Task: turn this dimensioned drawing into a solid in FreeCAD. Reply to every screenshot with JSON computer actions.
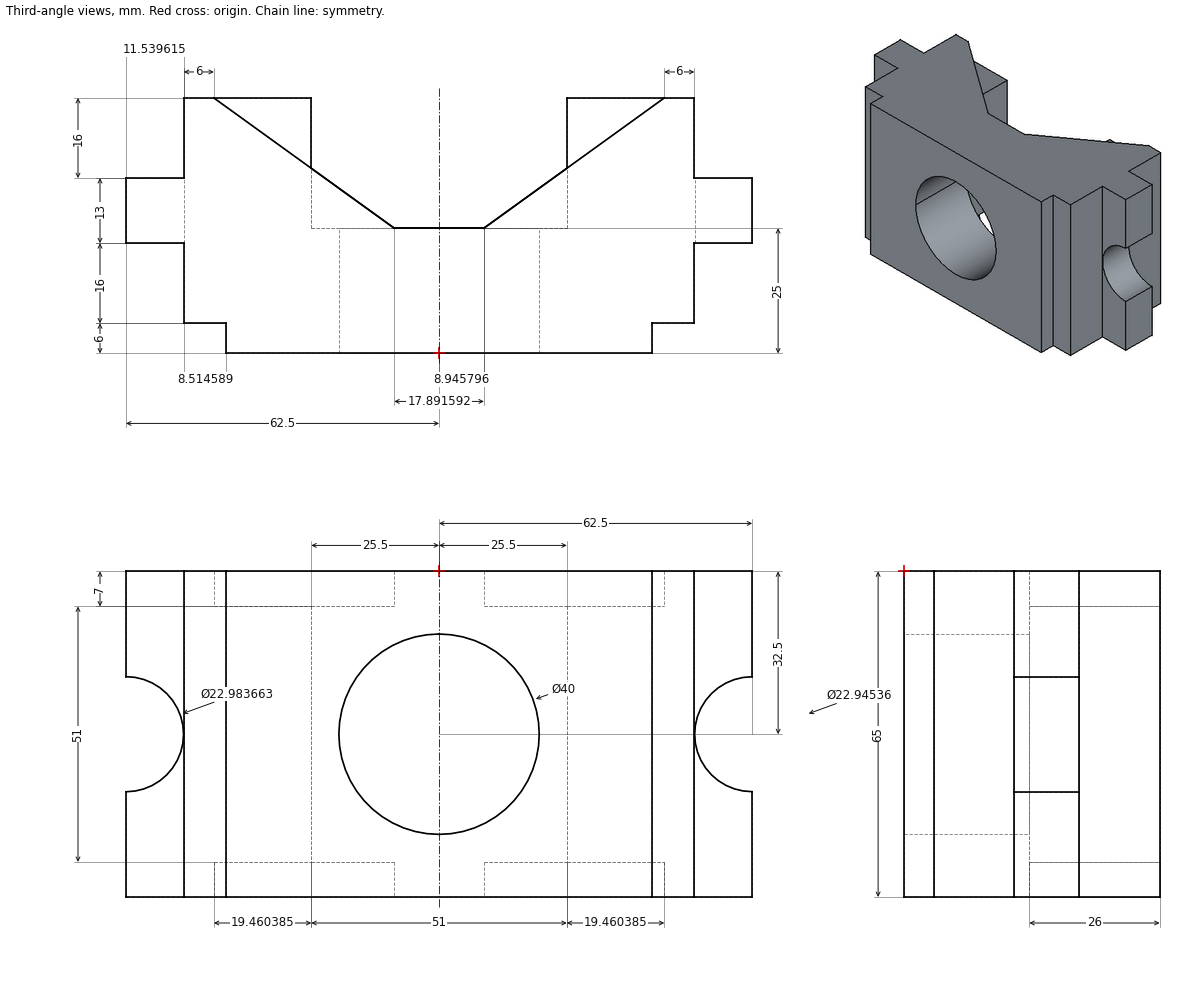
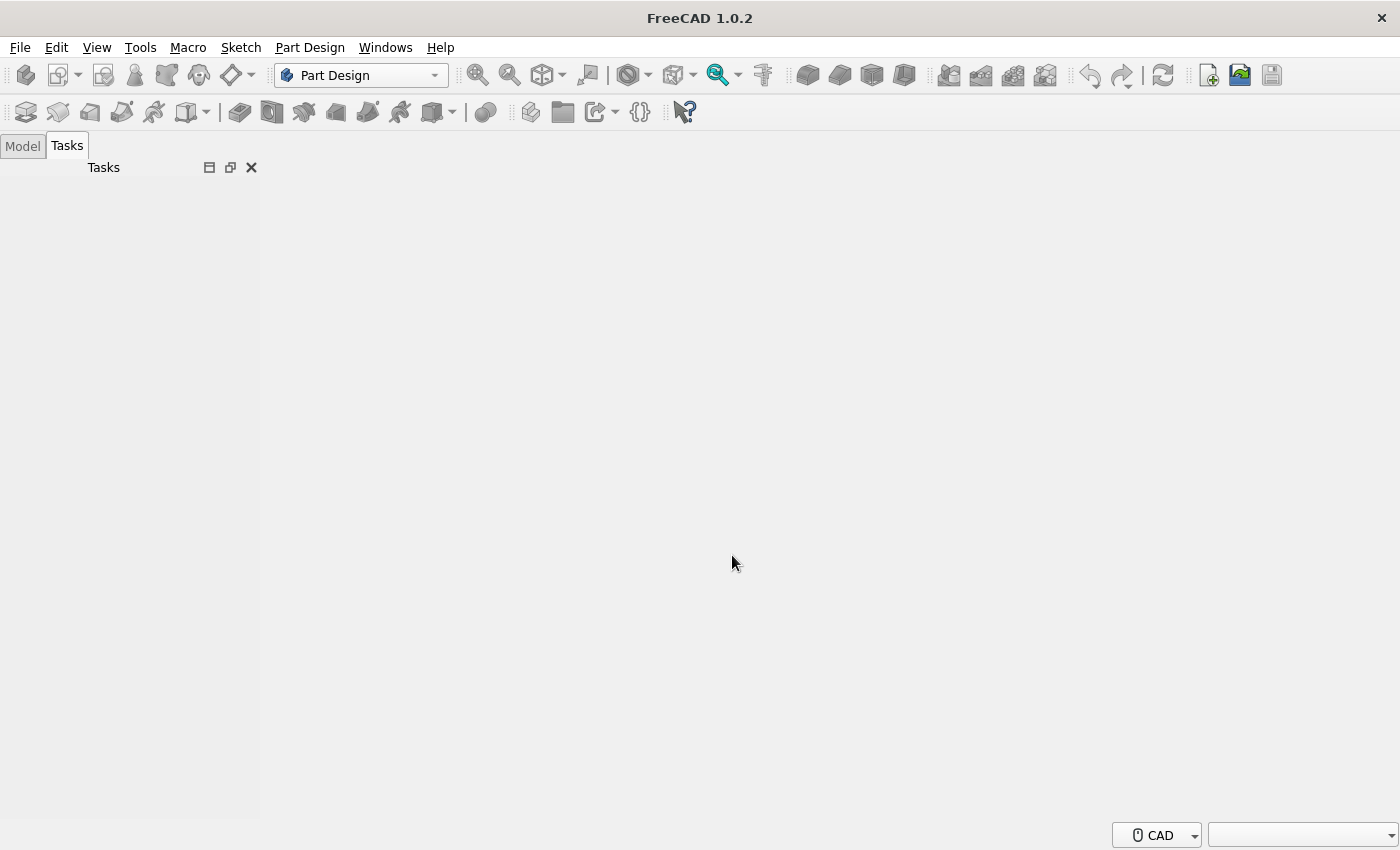
{"action": "left_click", "coordinate": [1208, 76]}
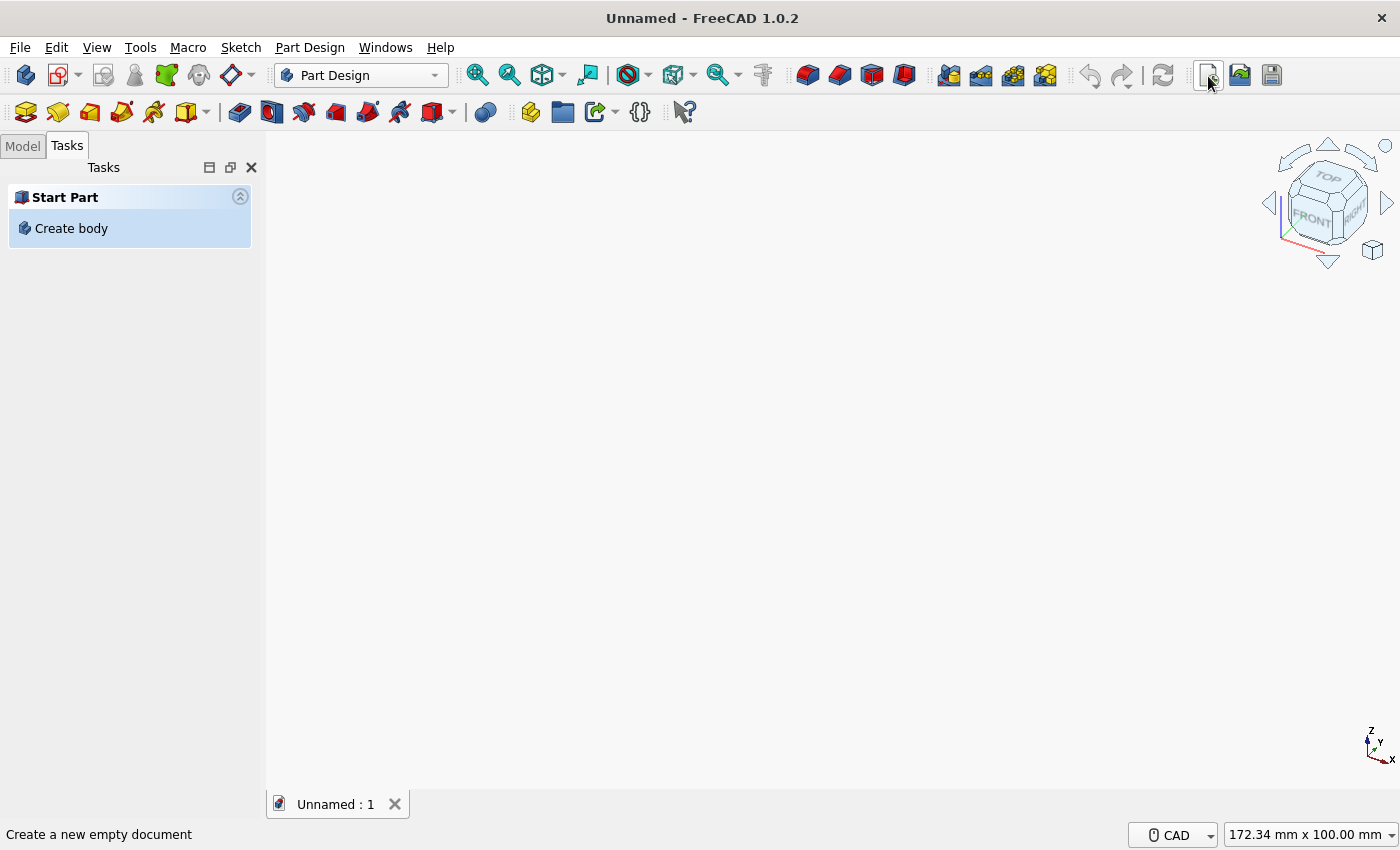
{"action": "left_click", "coordinate": [58, 76]}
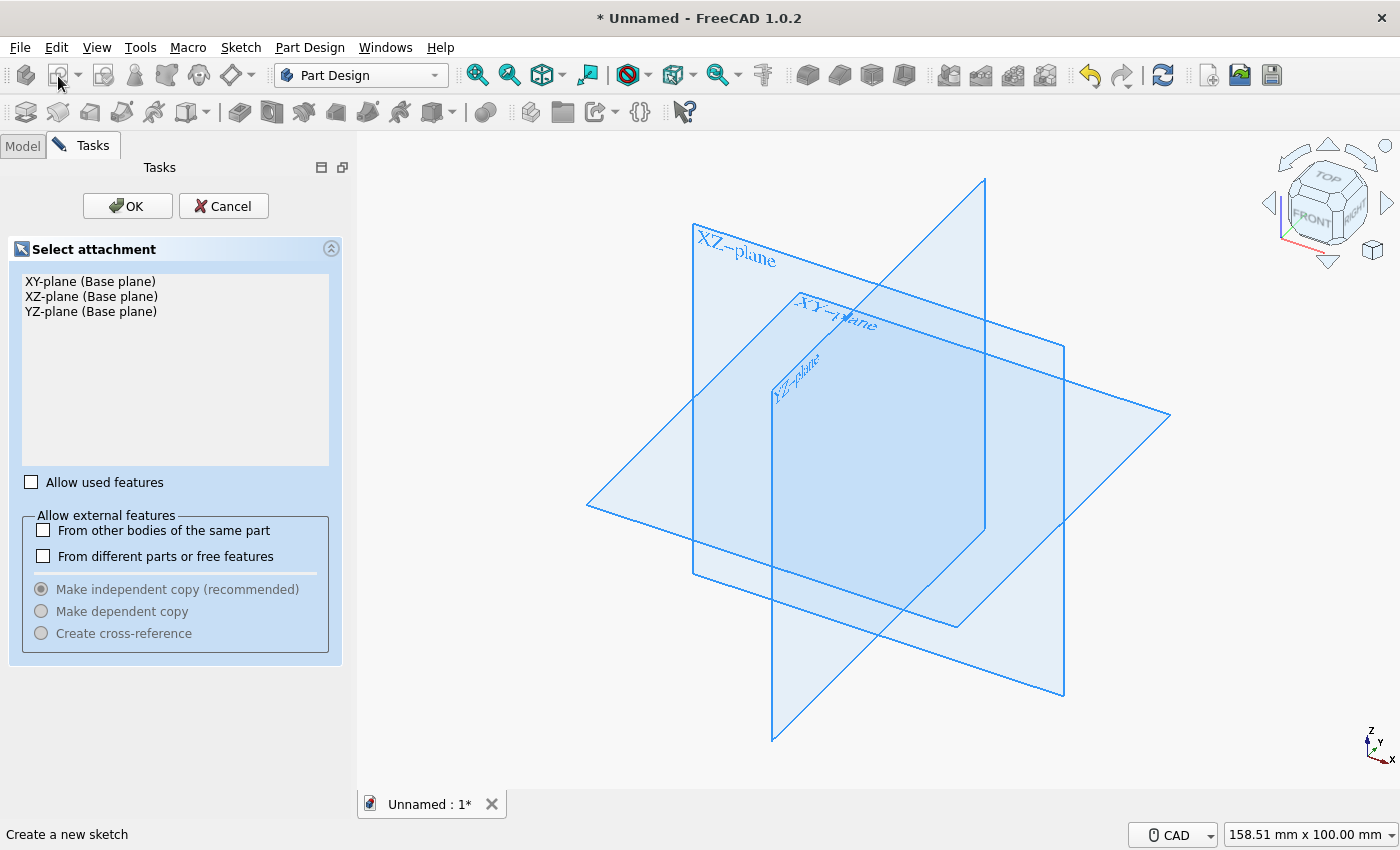
{"action": "left_click", "coordinate": [82, 282]}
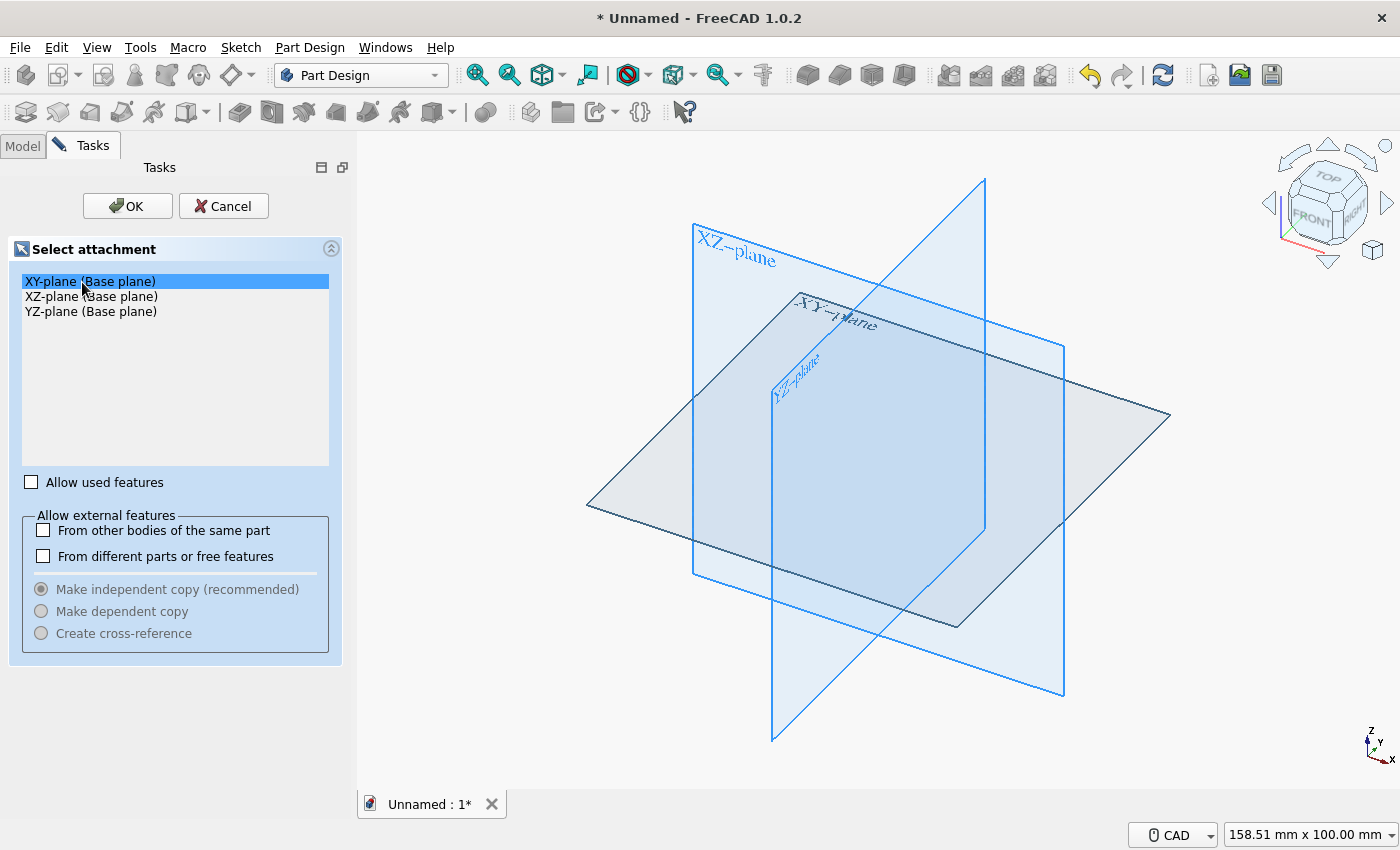
{"action": "left_click", "coordinate": [128, 206]}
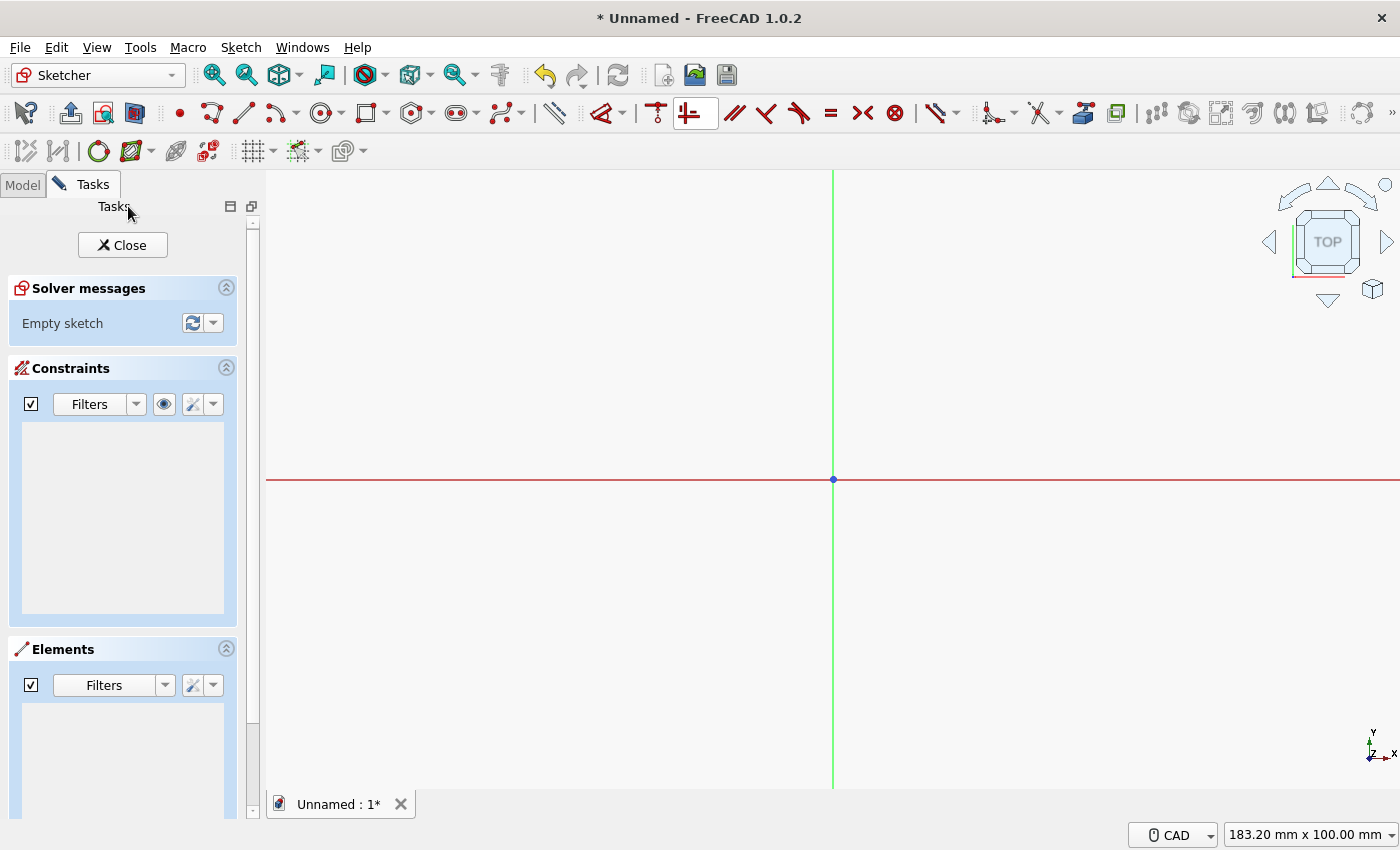
{"action": "scroll", "coordinate": [455, 761], "scroll_direction": "down", "scroll_amount": 1}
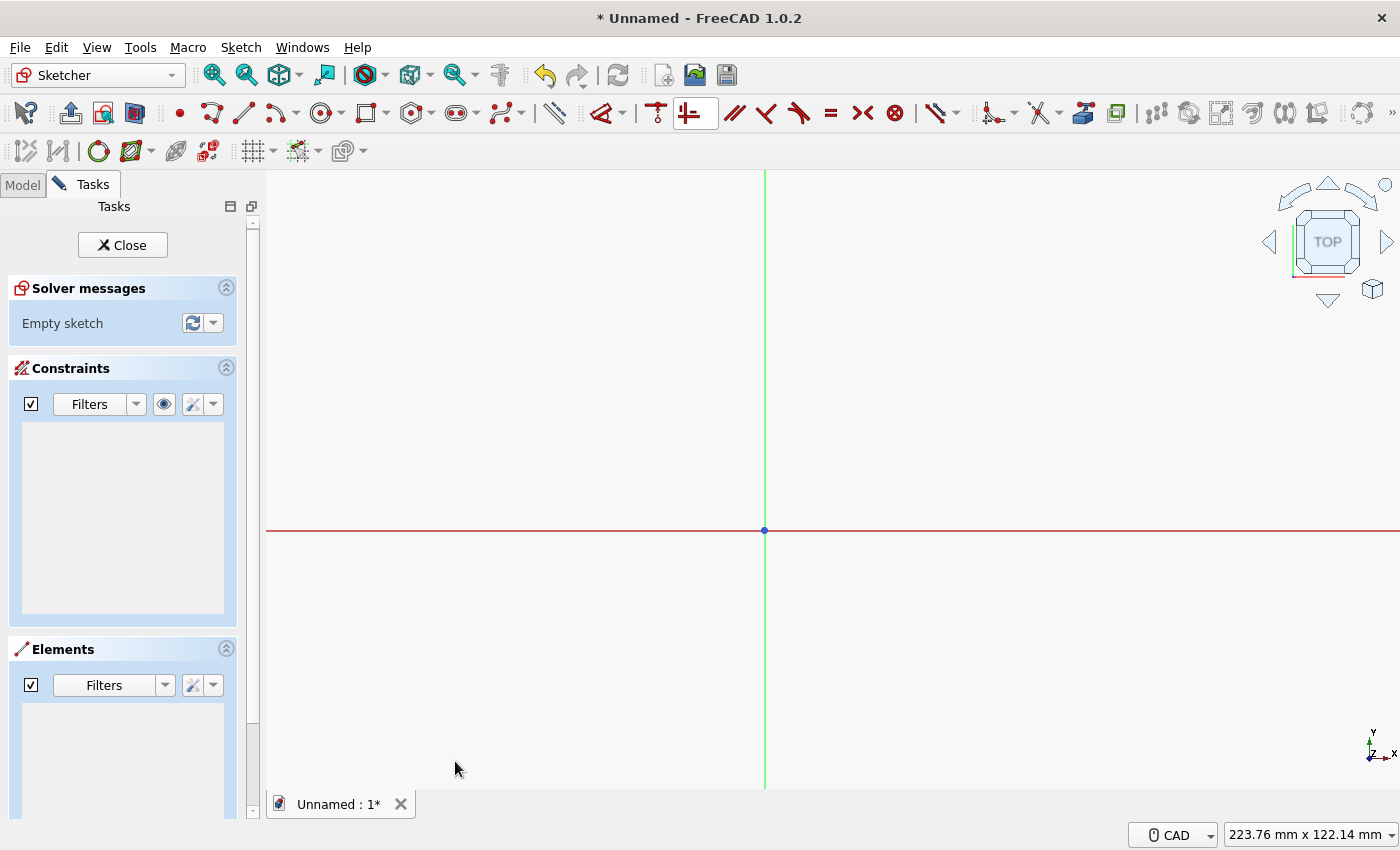
{"action": "left_click", "coordinate": [212, 114]}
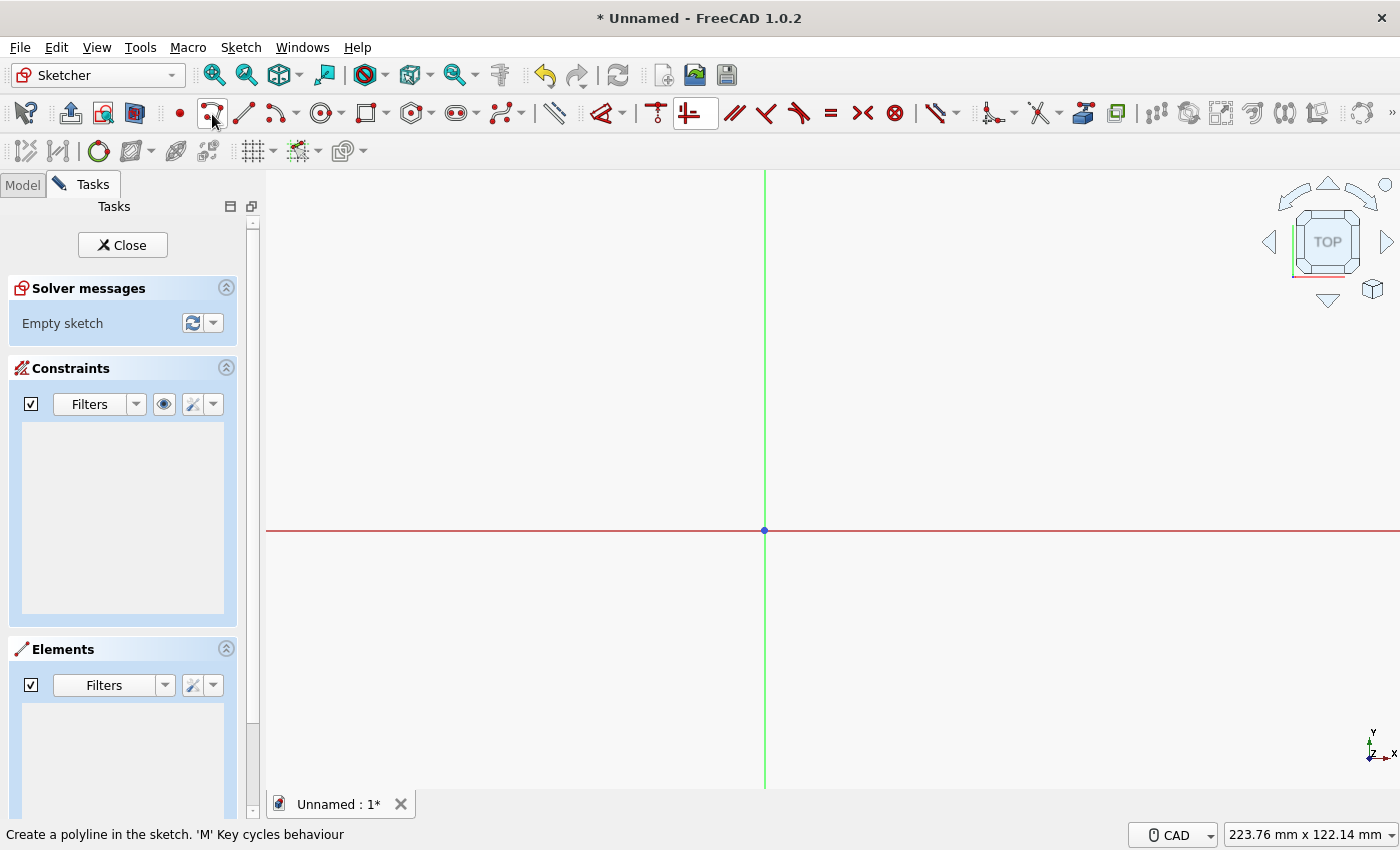
{"action": "left_click", "coordinate": [810, 404]}
{"action": "left_click", "coordinate": [719, 404]}
{"action": "left_click", "coordinate": [537, 272]}
{"action": "left_click", "coordinate": [506, 272]}
{"action": "left_click", "coordinate": [506, 353]}
{"action": "left_click", "coordinate": [448, 353]}
{"action": "left_click", "coordinate": [448, 419]}
{"action": "left_click", "coordinate": [506, 419]}
{"action": "left_click", "coordinate": [506, 500]}
{"action": "left_click", "coordinate": [549, 500]}
{"action": "left_click", "coordinate": [549, 531]}
{"action": "left_click", "coordinate": [980, 522]}
{"action": "left_click", "coordinate": [980, 500]}
{"action": "left_click", "coordinate": [1023, 500]}
{"action": "left_click", "coordinate": [1023, 419]}
{"action": "left_click", "coordinate": [1081, 419]}
{"action": "left_click", "coordinate": [1081, 353]}
{"action": "left_click", "coordinate": [1023, 353]}
{"action": "left_click", "coordinate": [1023, 272]}
{"action": "left_click", "coordinate": [992, 272]}
{"action": "left_click", "coordinate": [810, 405]}
{"action": "key", "text": "Escape"}
{"action": "key", "text": "Escape"}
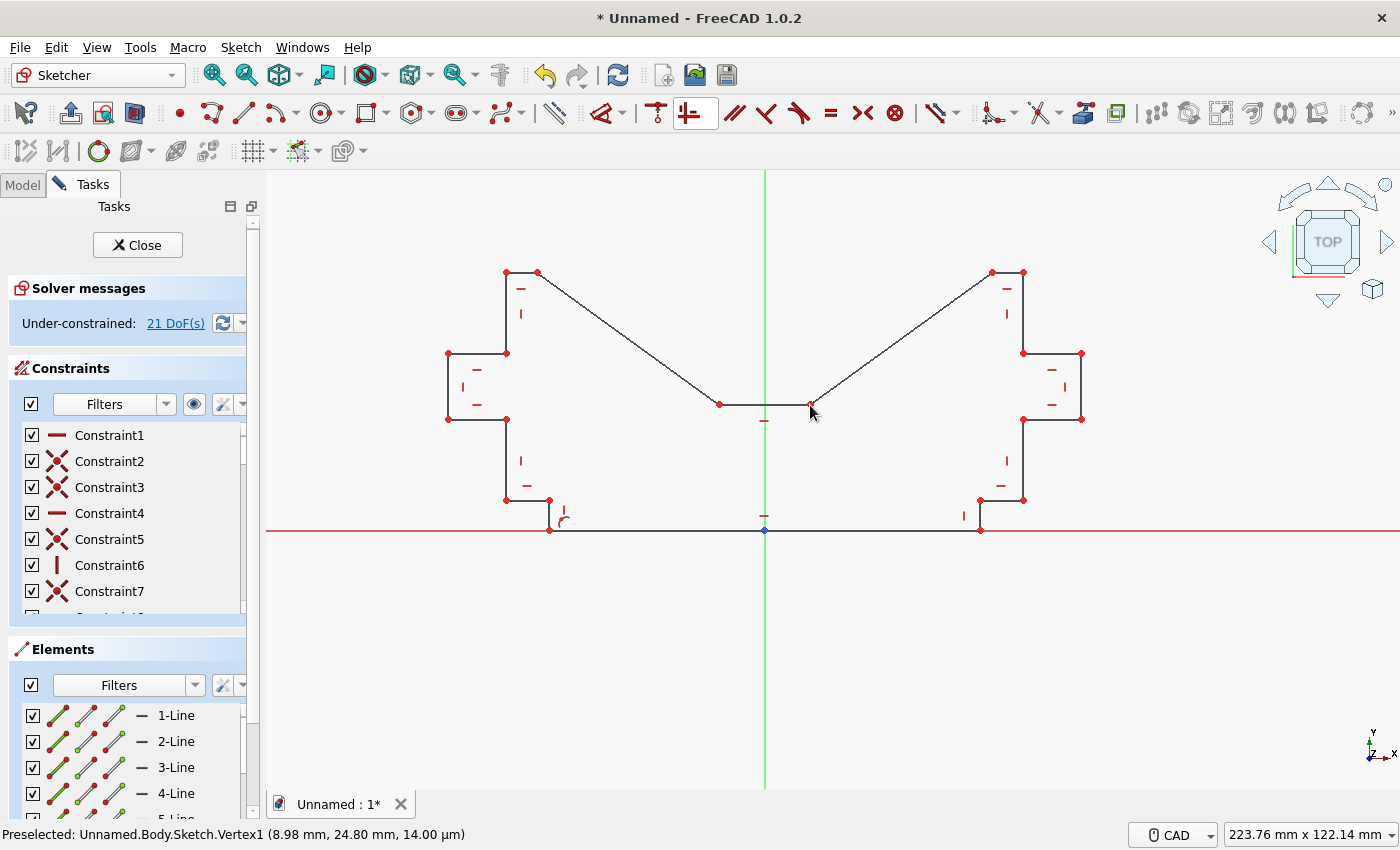
{"action": "left_click", "coordinate": [549, 501]}